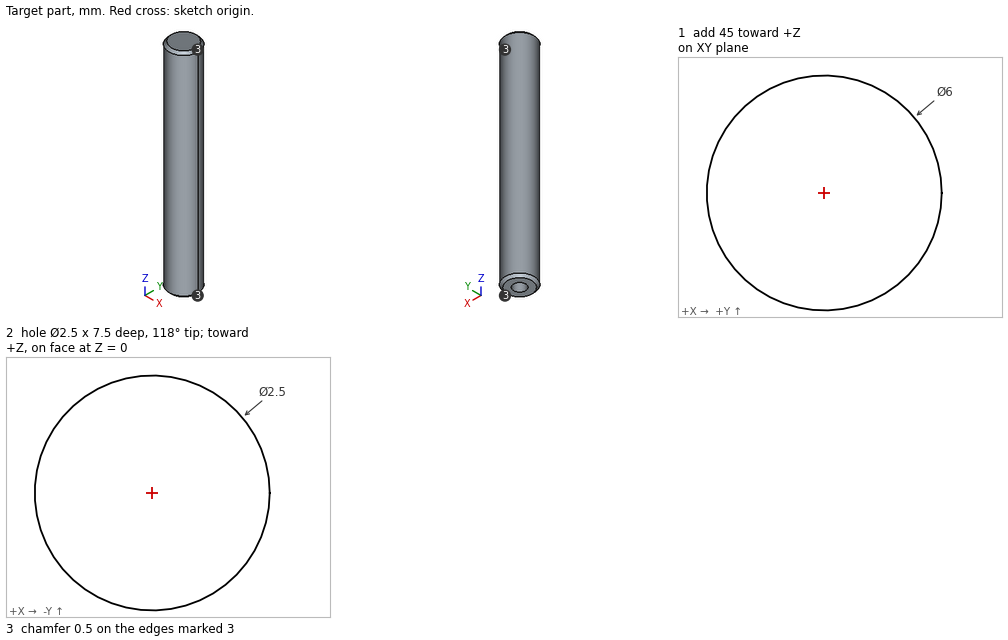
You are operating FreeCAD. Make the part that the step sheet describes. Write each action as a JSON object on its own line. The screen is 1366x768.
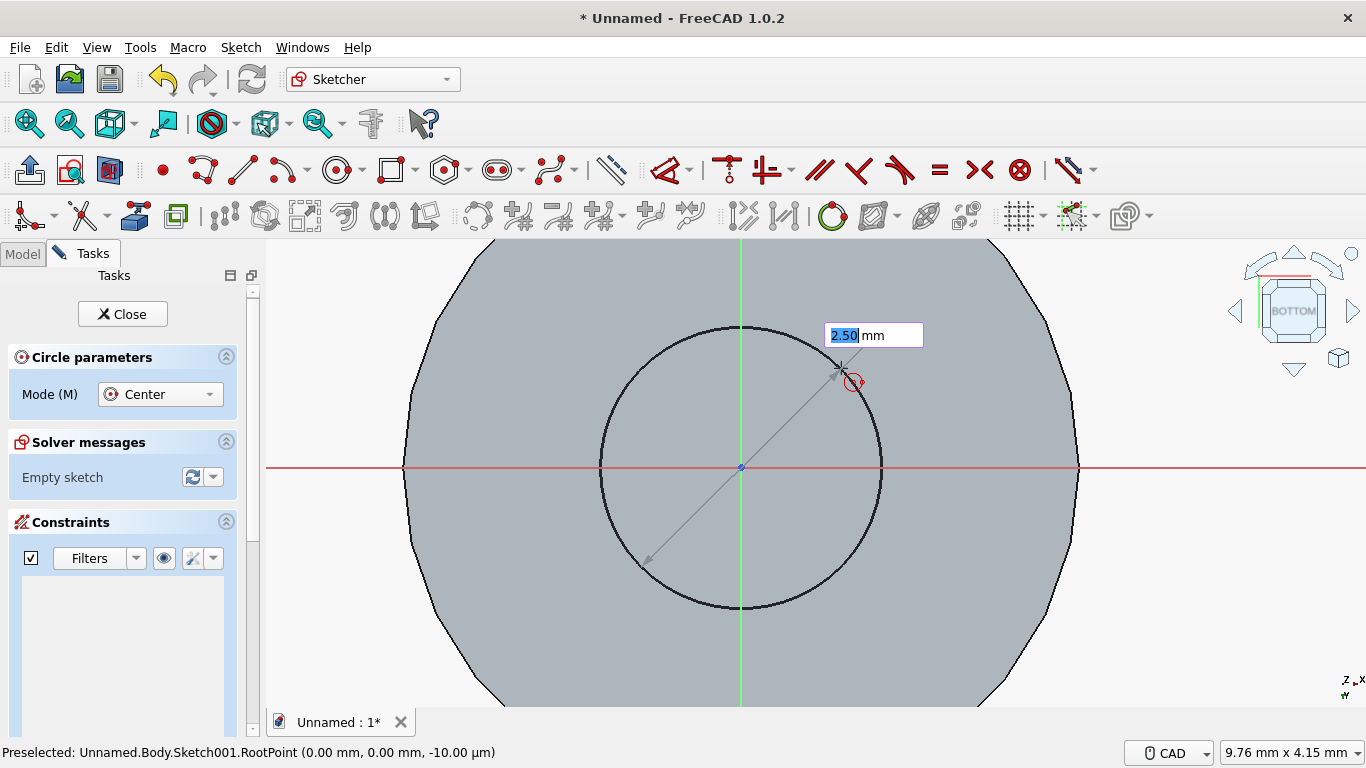
{"action": "type", "text": "2.5"}
{"action": "key", "text": "Return"}
{"action": "key", "text": "Escape"}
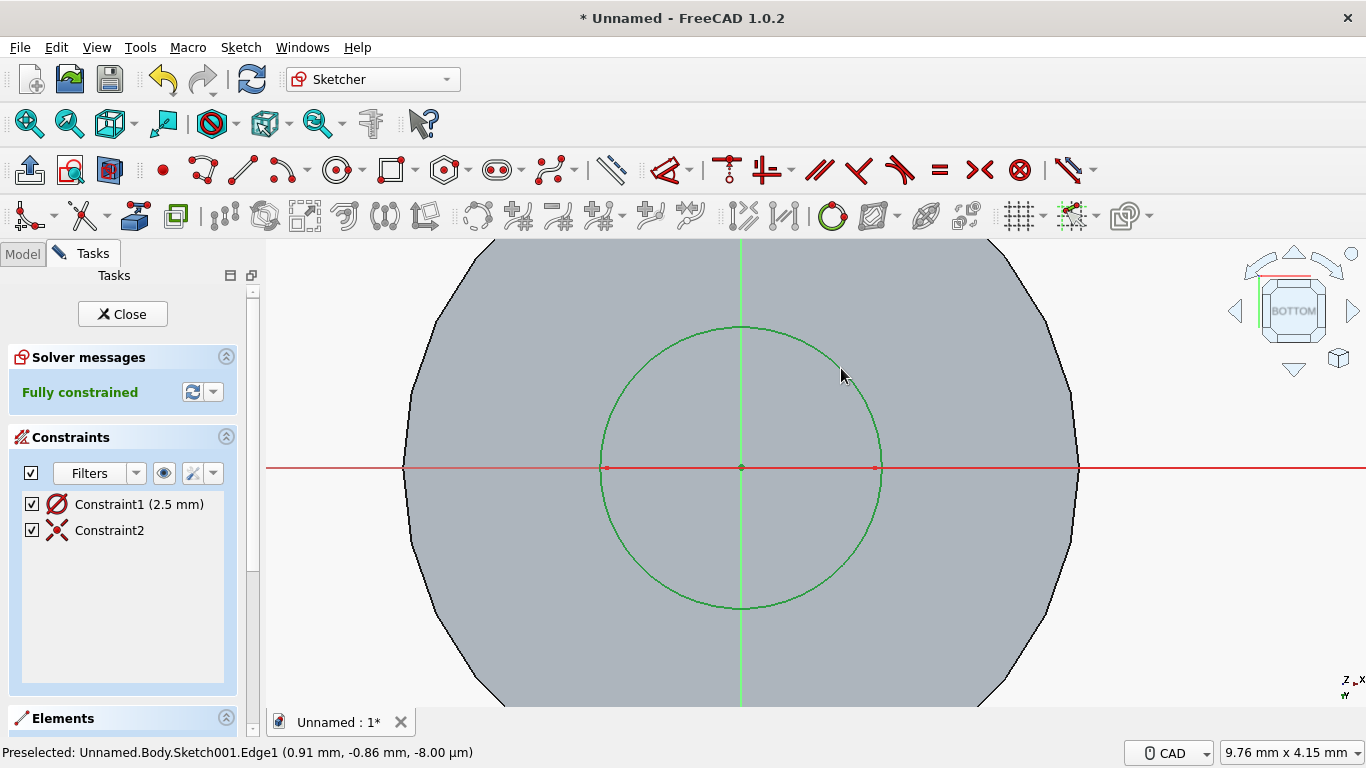
{"action": "left_click", "coordinate": [123, 314]}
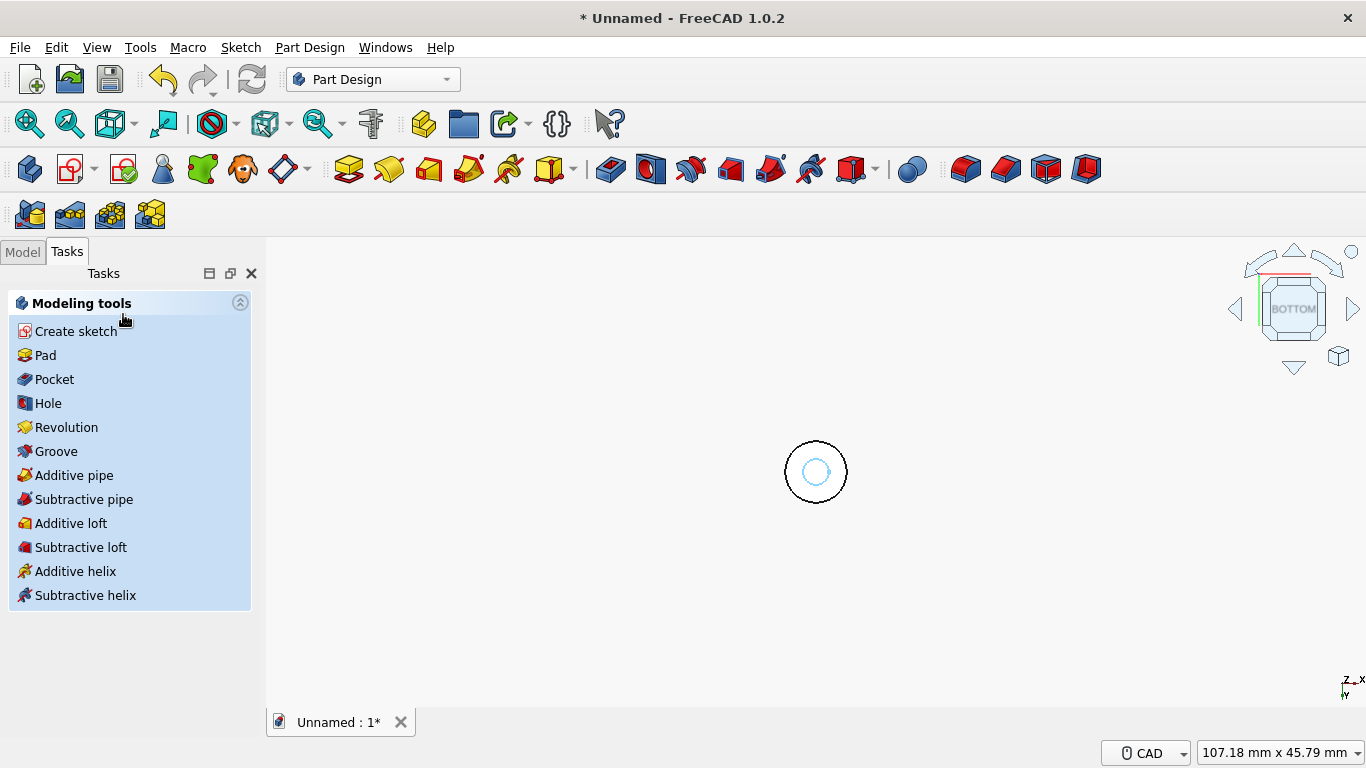
{"action": "left_click", "coordinate": [652, 170]}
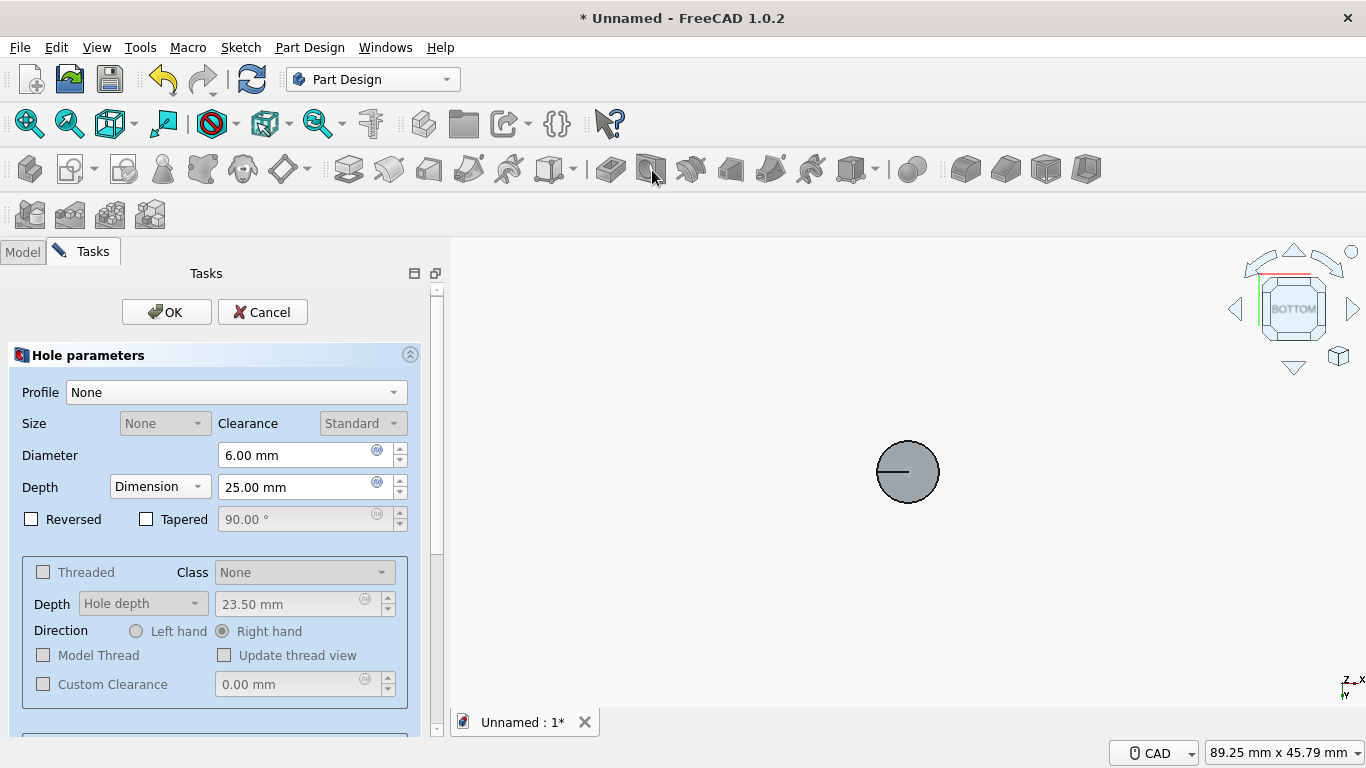
{"action": "triple_click", "coordinate": [305, 455]}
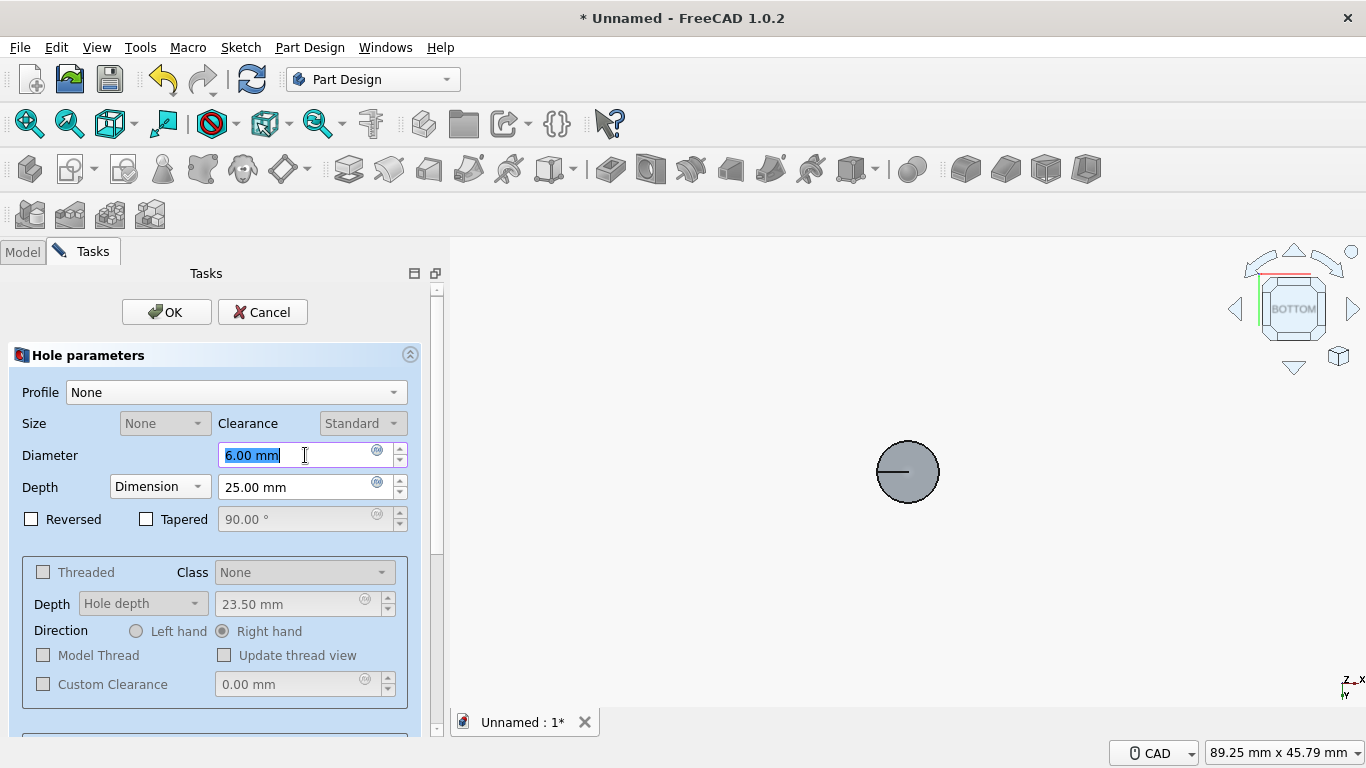
{"action": "type", "text": "2.5"}
{"action": "key", "text": "Tab"}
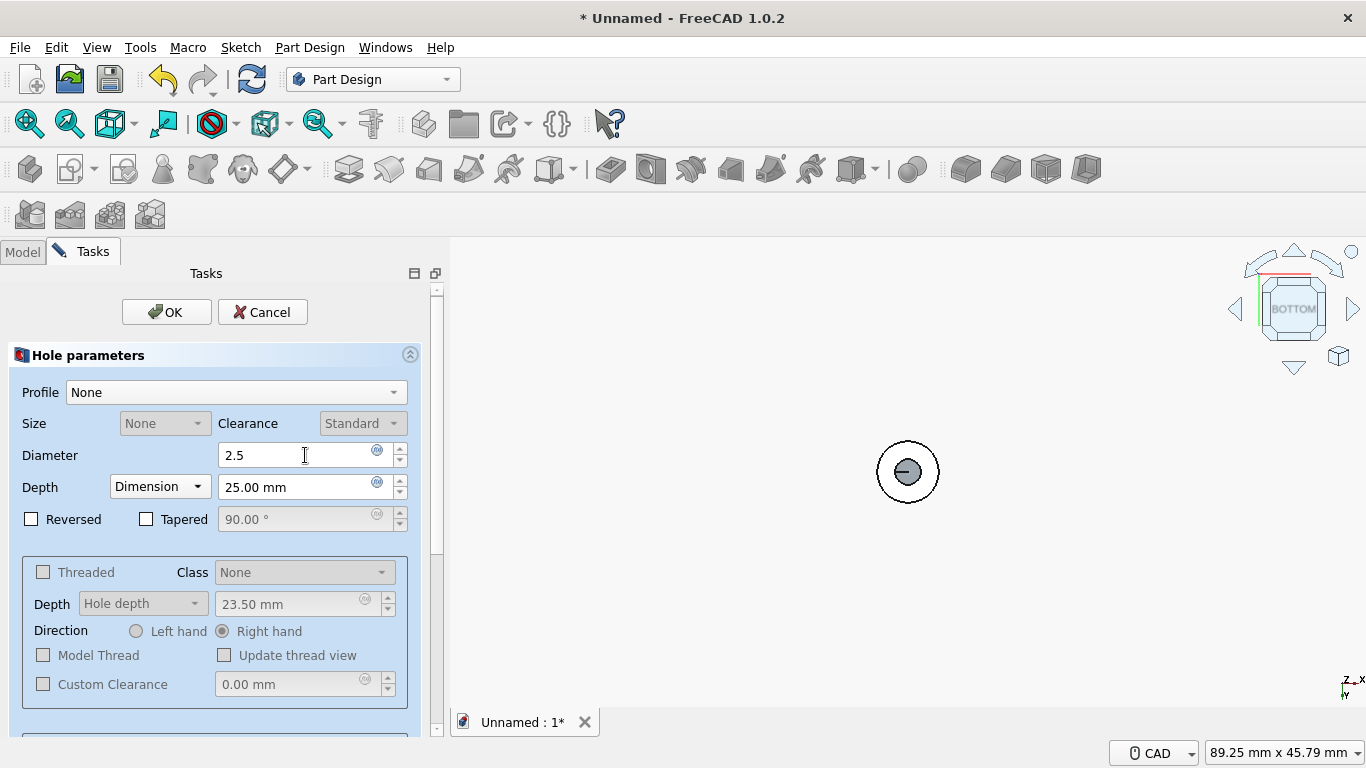
{"action": "triple_click", "coordinate": [305, 487]}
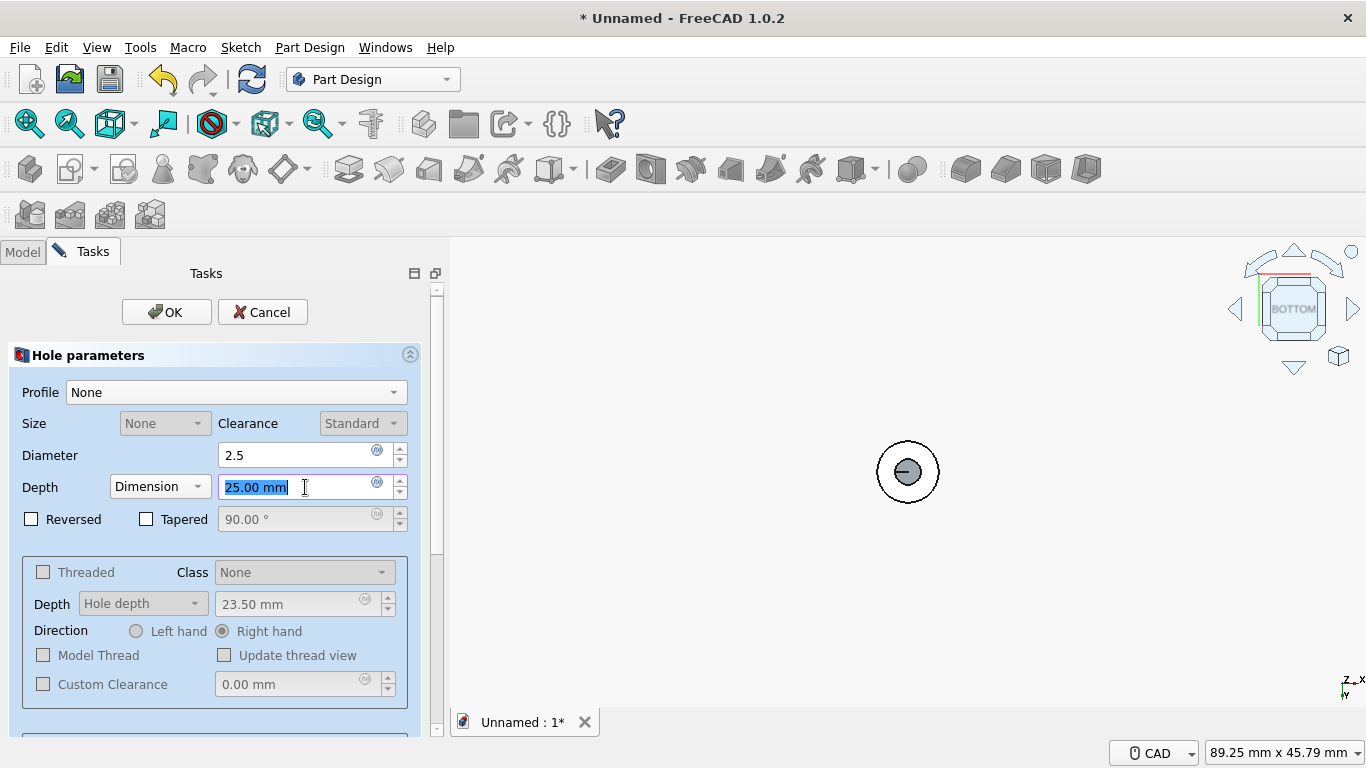
{"action": "type", "text": "7.5"}
{"action": "key", "text": "Tab"}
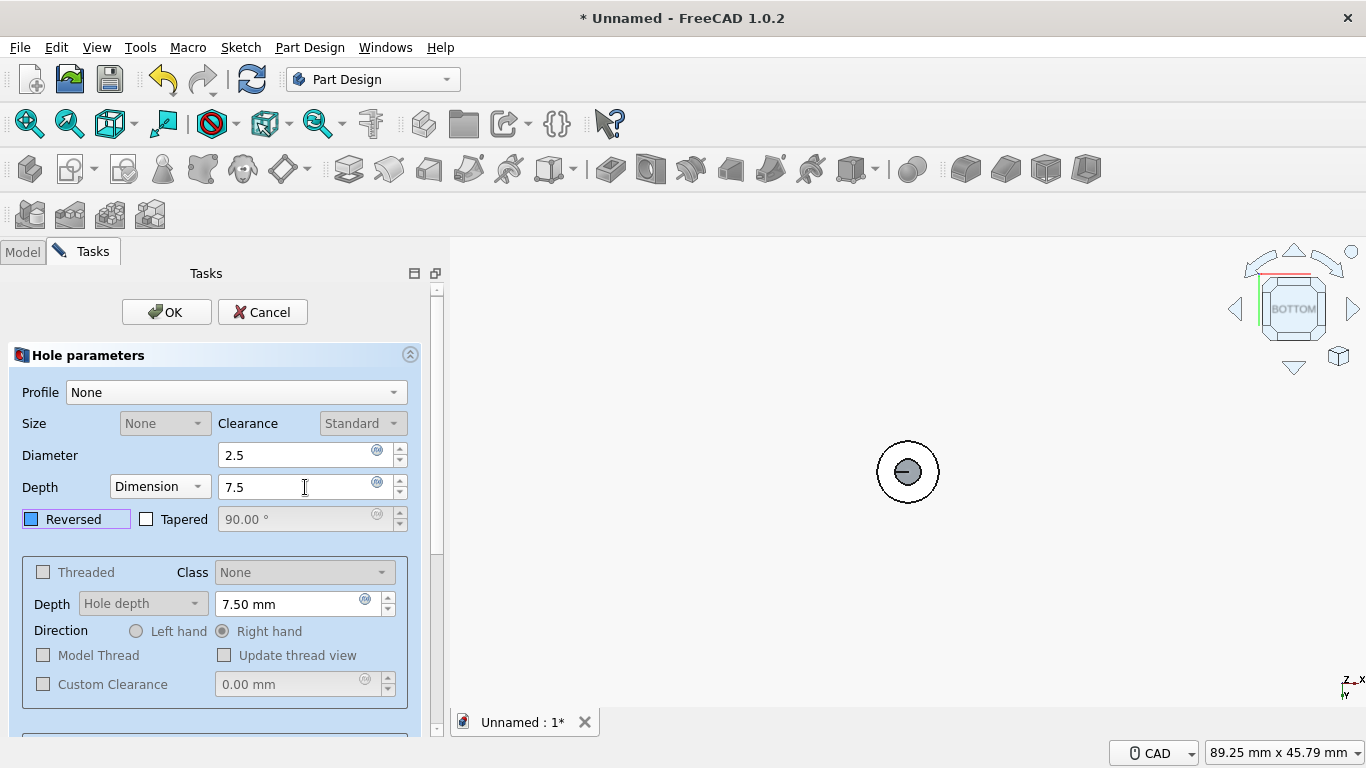
{"action": "left_click", "coordinate": [167, 312]}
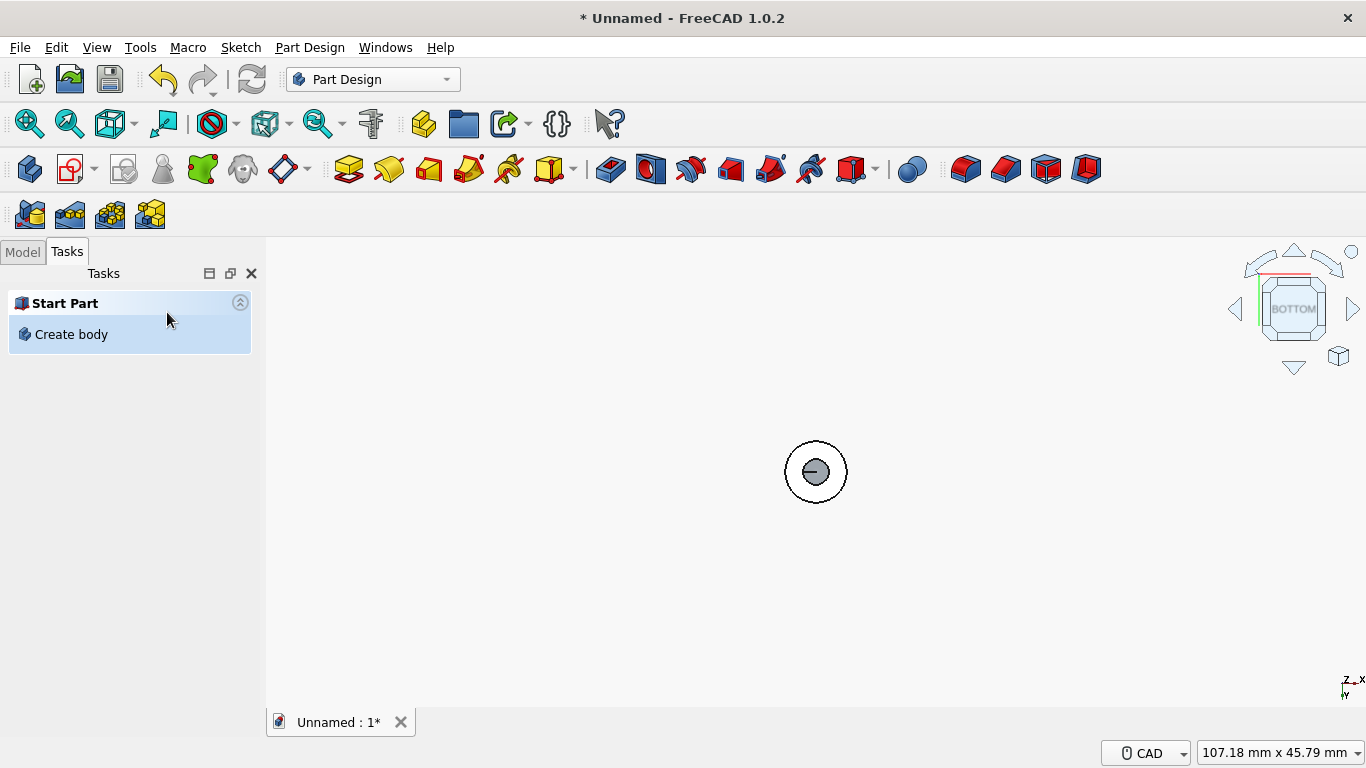
{"action": "left_click", "coordinate": [30, 124]}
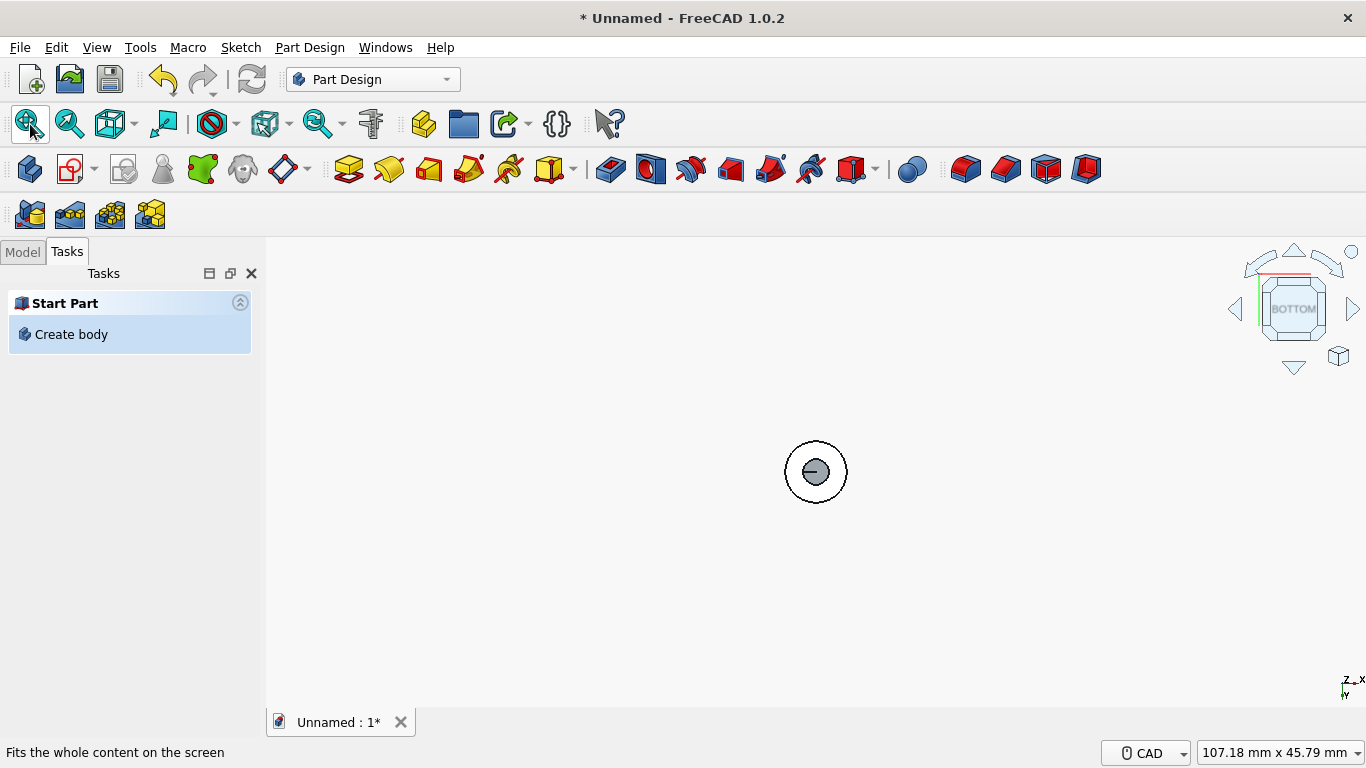
{"action": "left_click", "coordinate": [785, 471]}